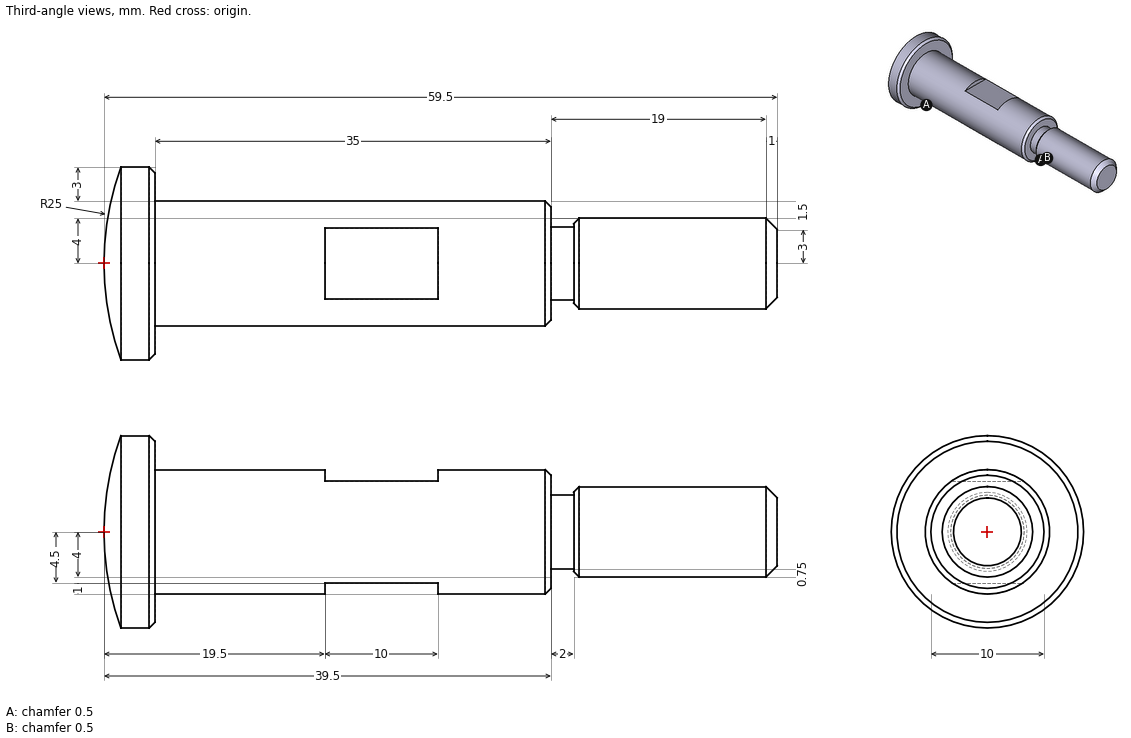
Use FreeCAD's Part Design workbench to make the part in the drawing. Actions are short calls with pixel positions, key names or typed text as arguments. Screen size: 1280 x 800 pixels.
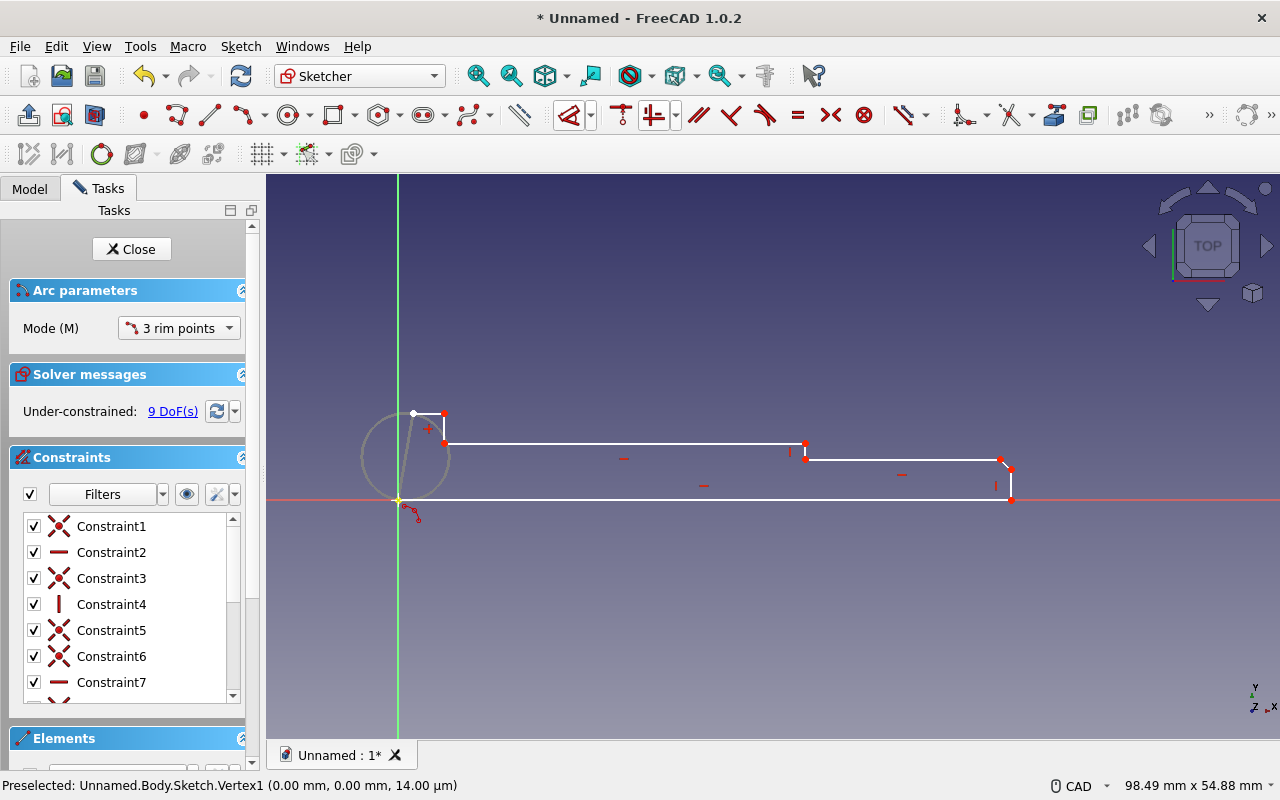
scroll(402, 456, up, 8)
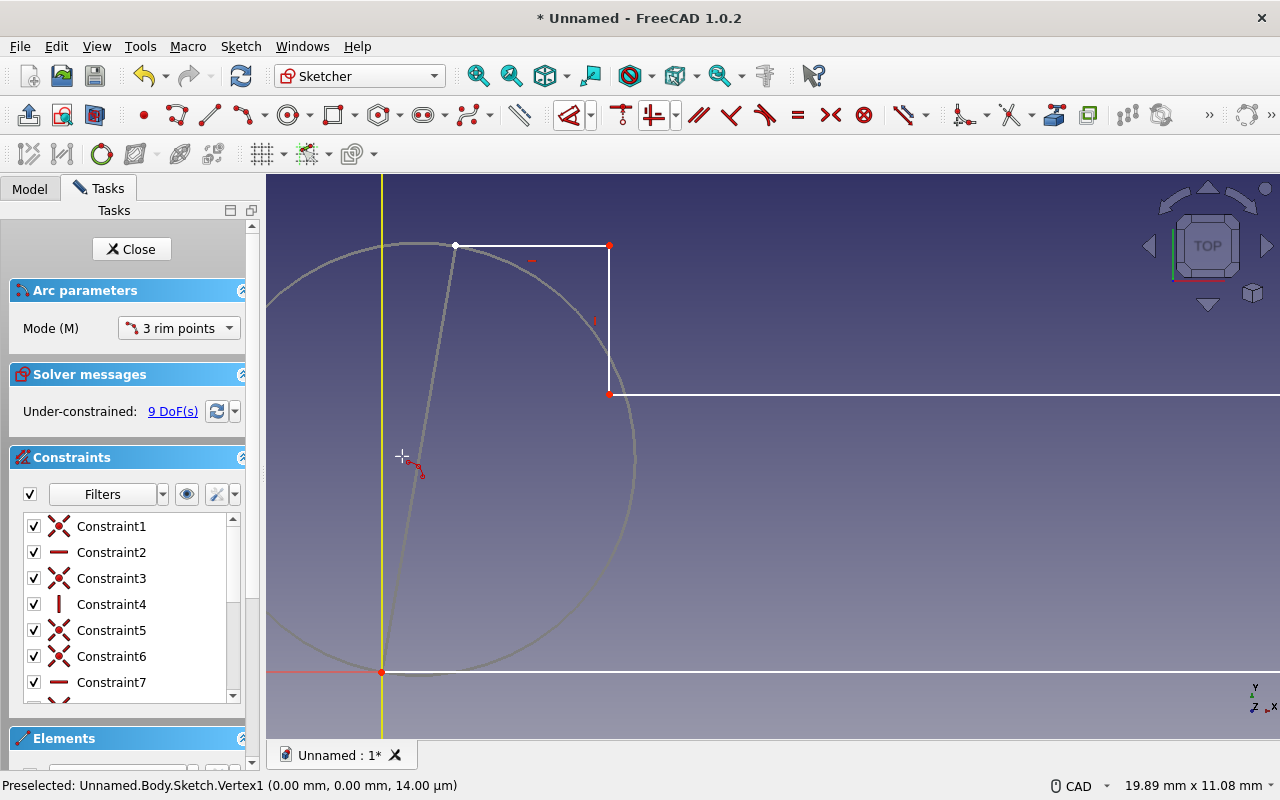
click(401, 452)
key(Escape)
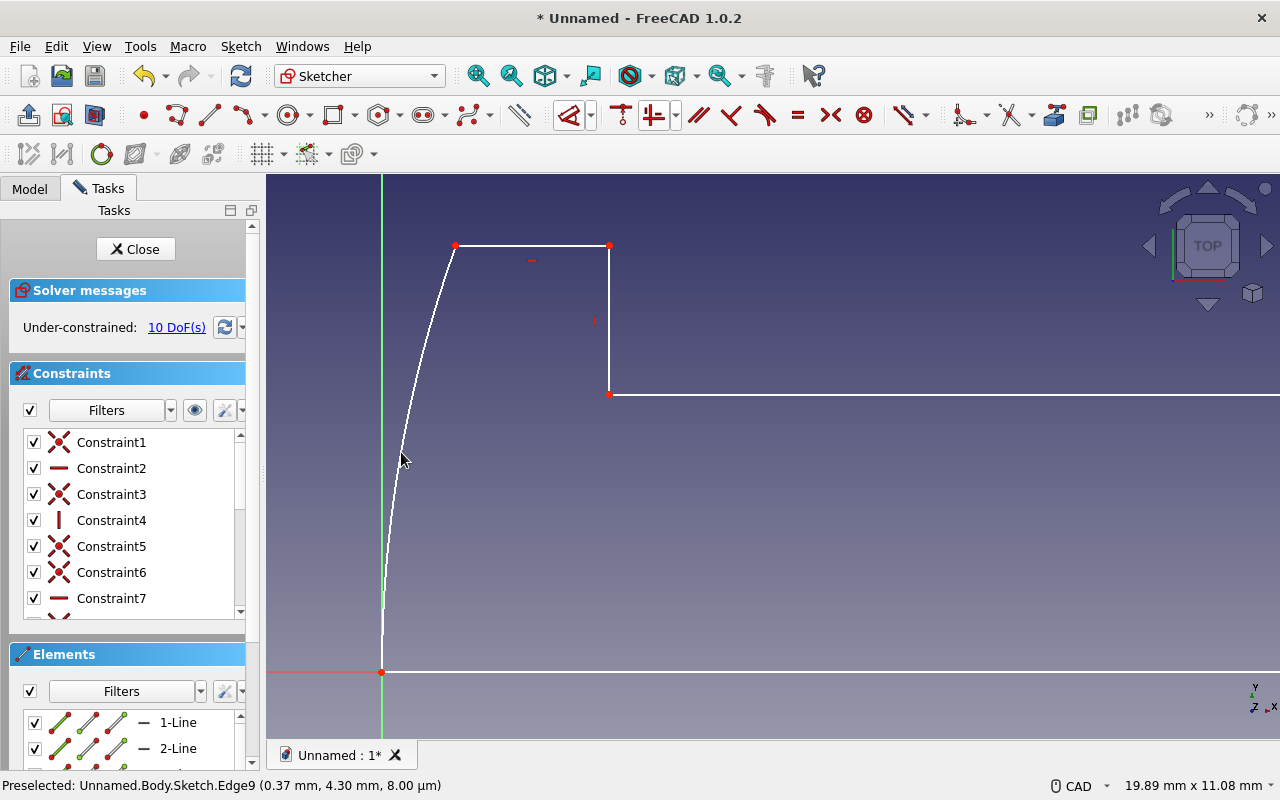
scroll(402, 457, down, 8)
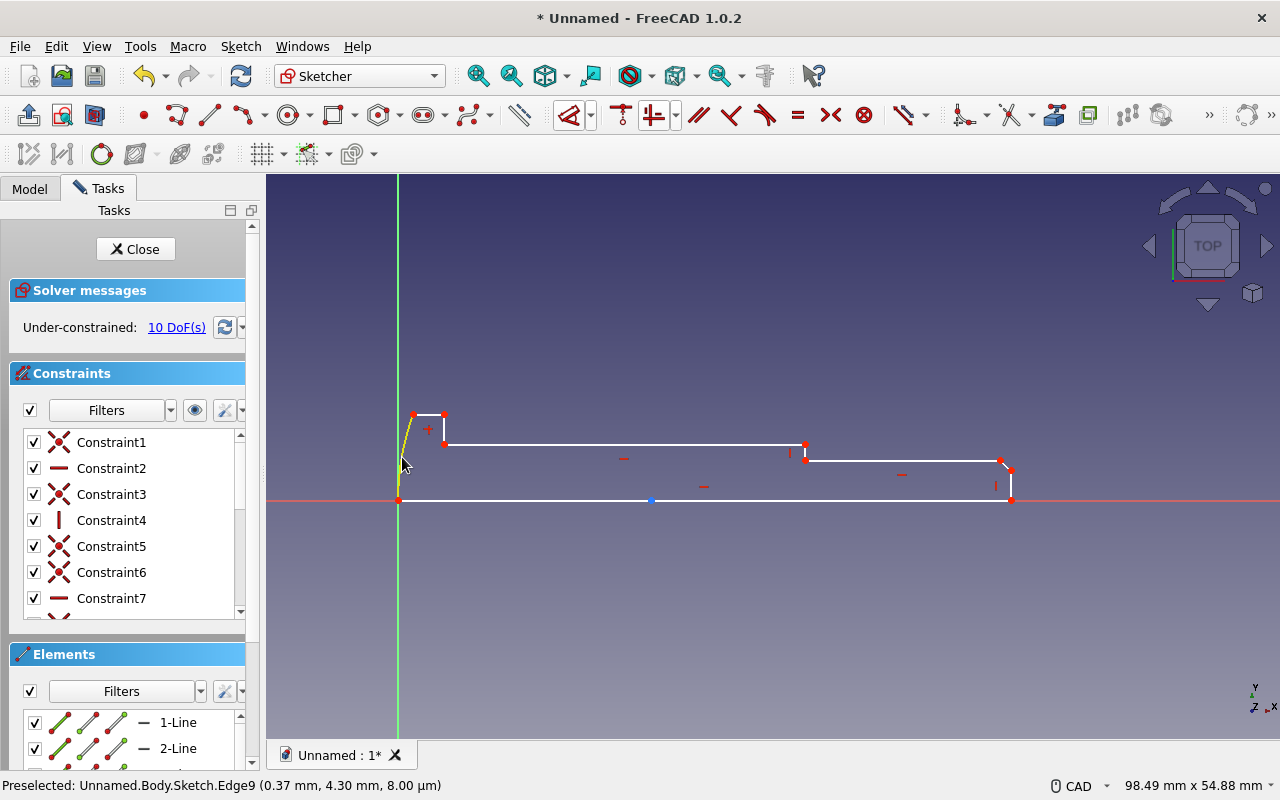
click(652, 501)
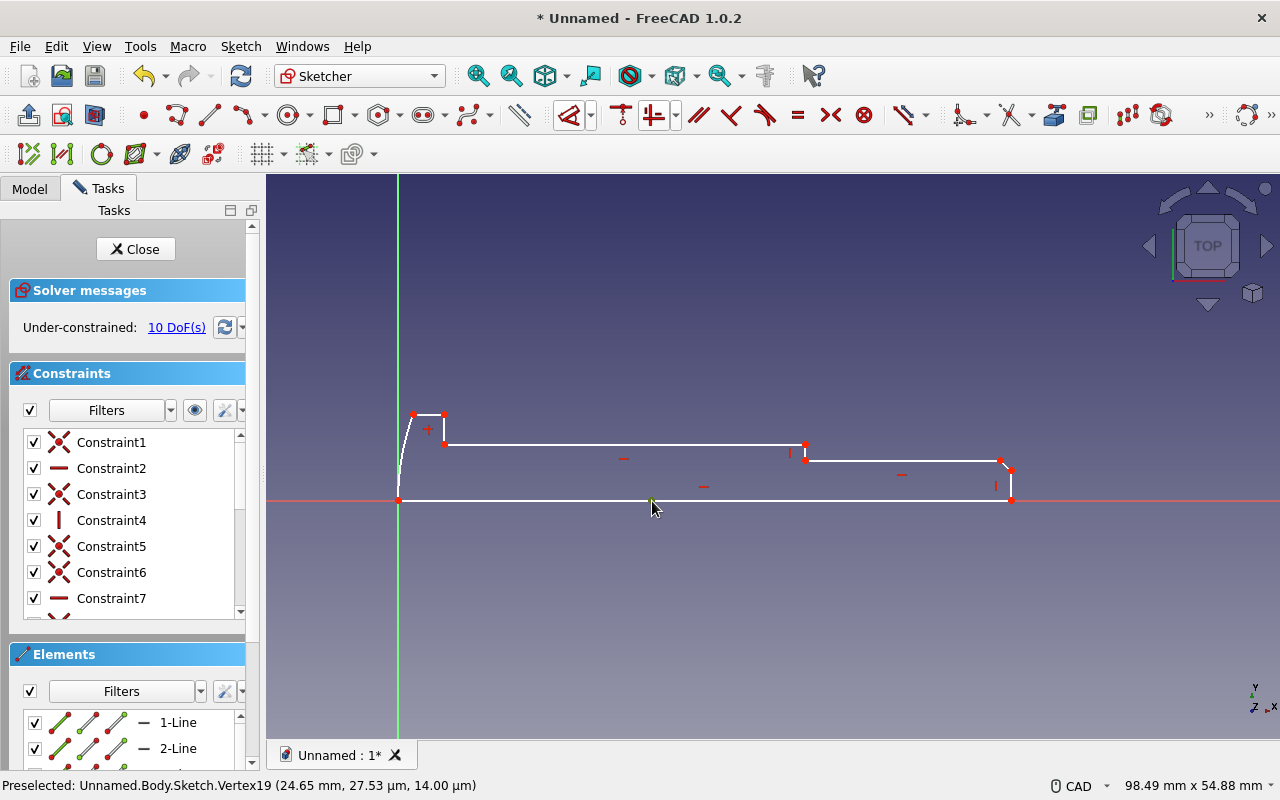
click(353, 501)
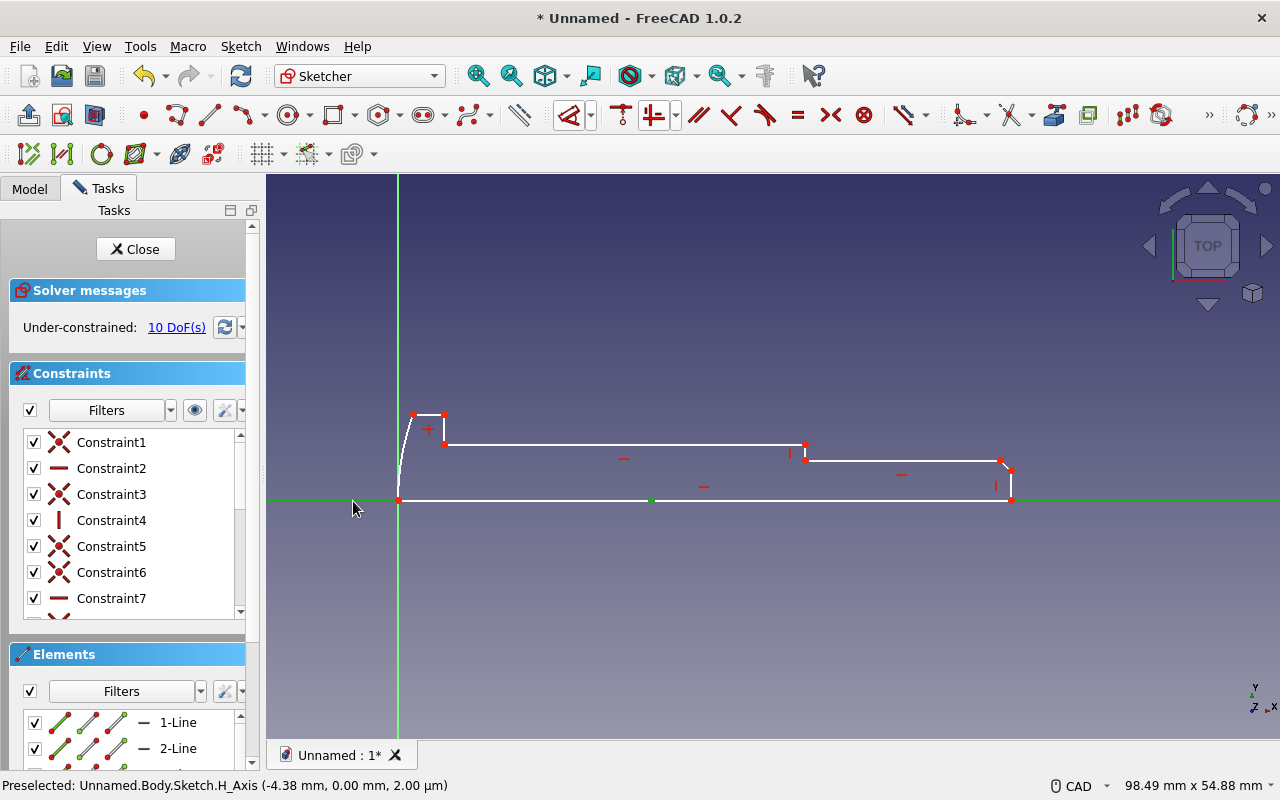
key(c)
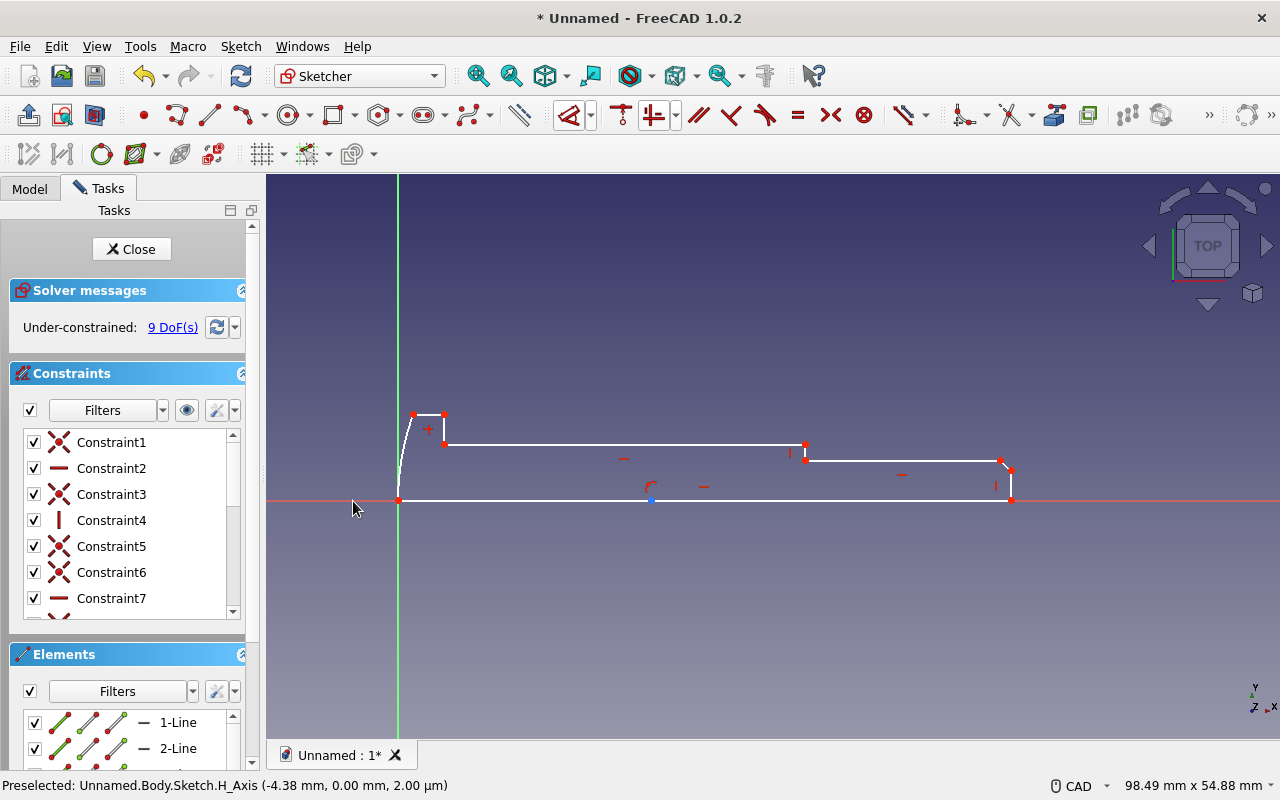
click(568, 116)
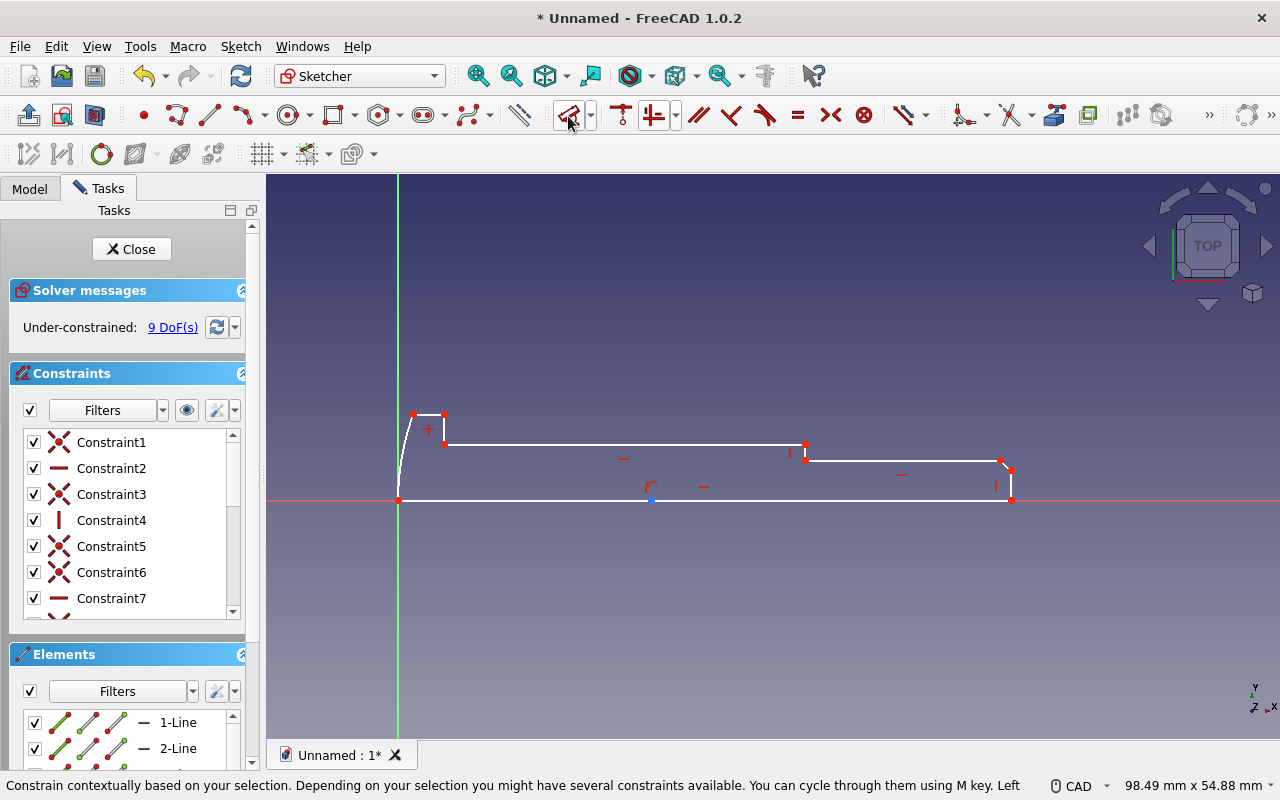
click(399, 475)
click(367, 472)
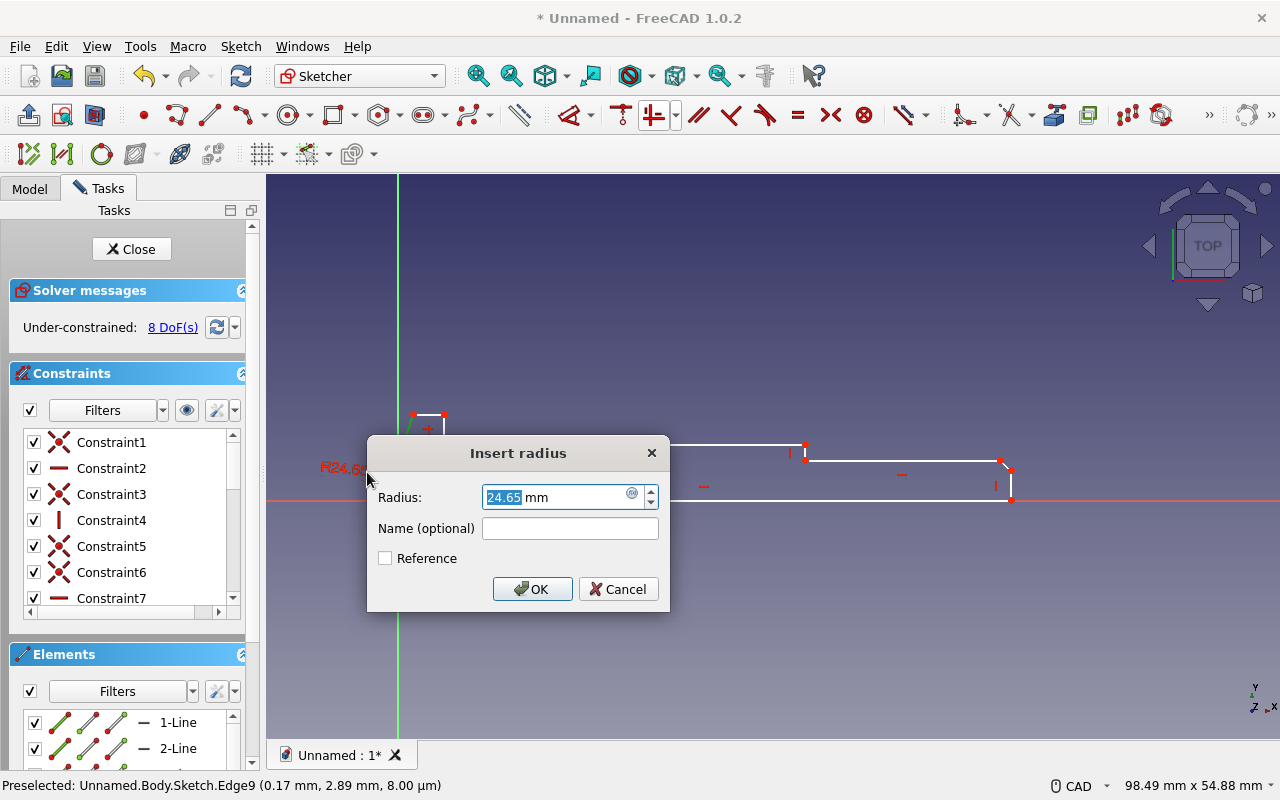
text(25)
key(Return)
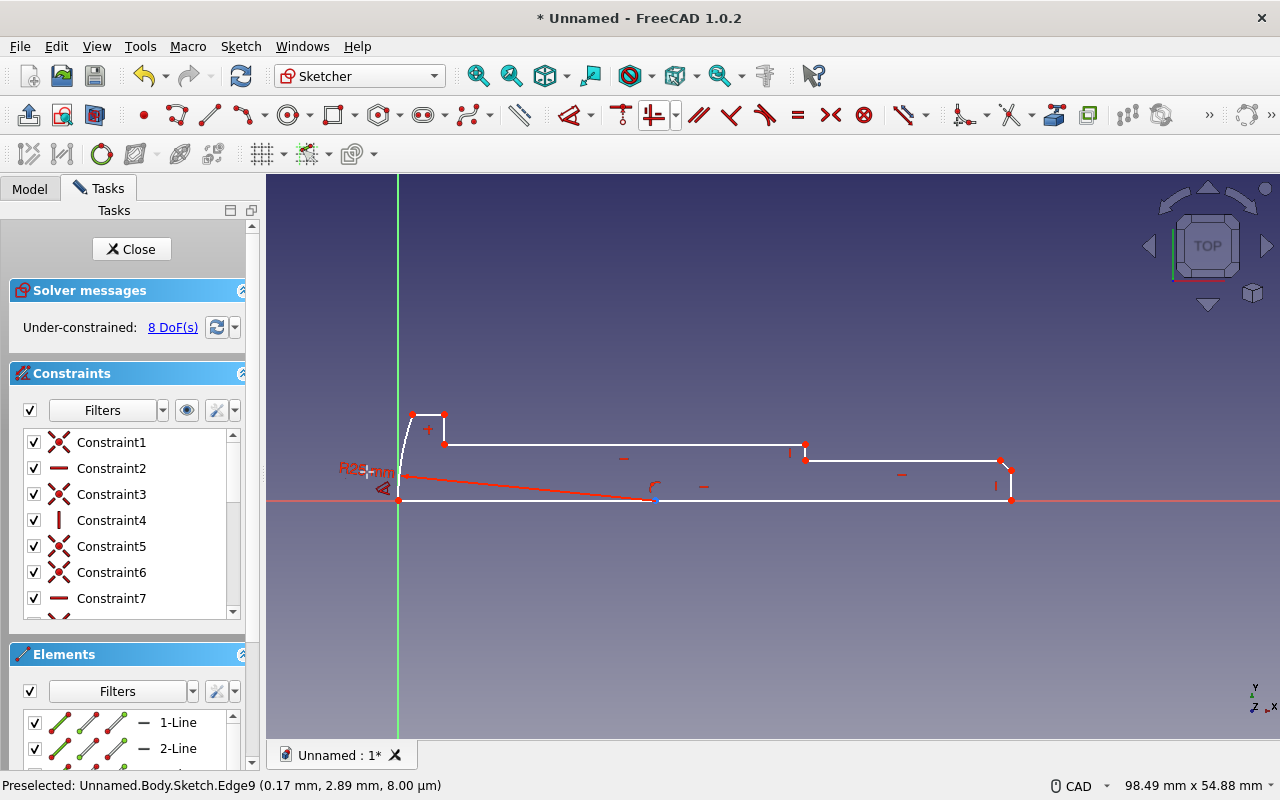
scroll(1011, 492, up, 3)